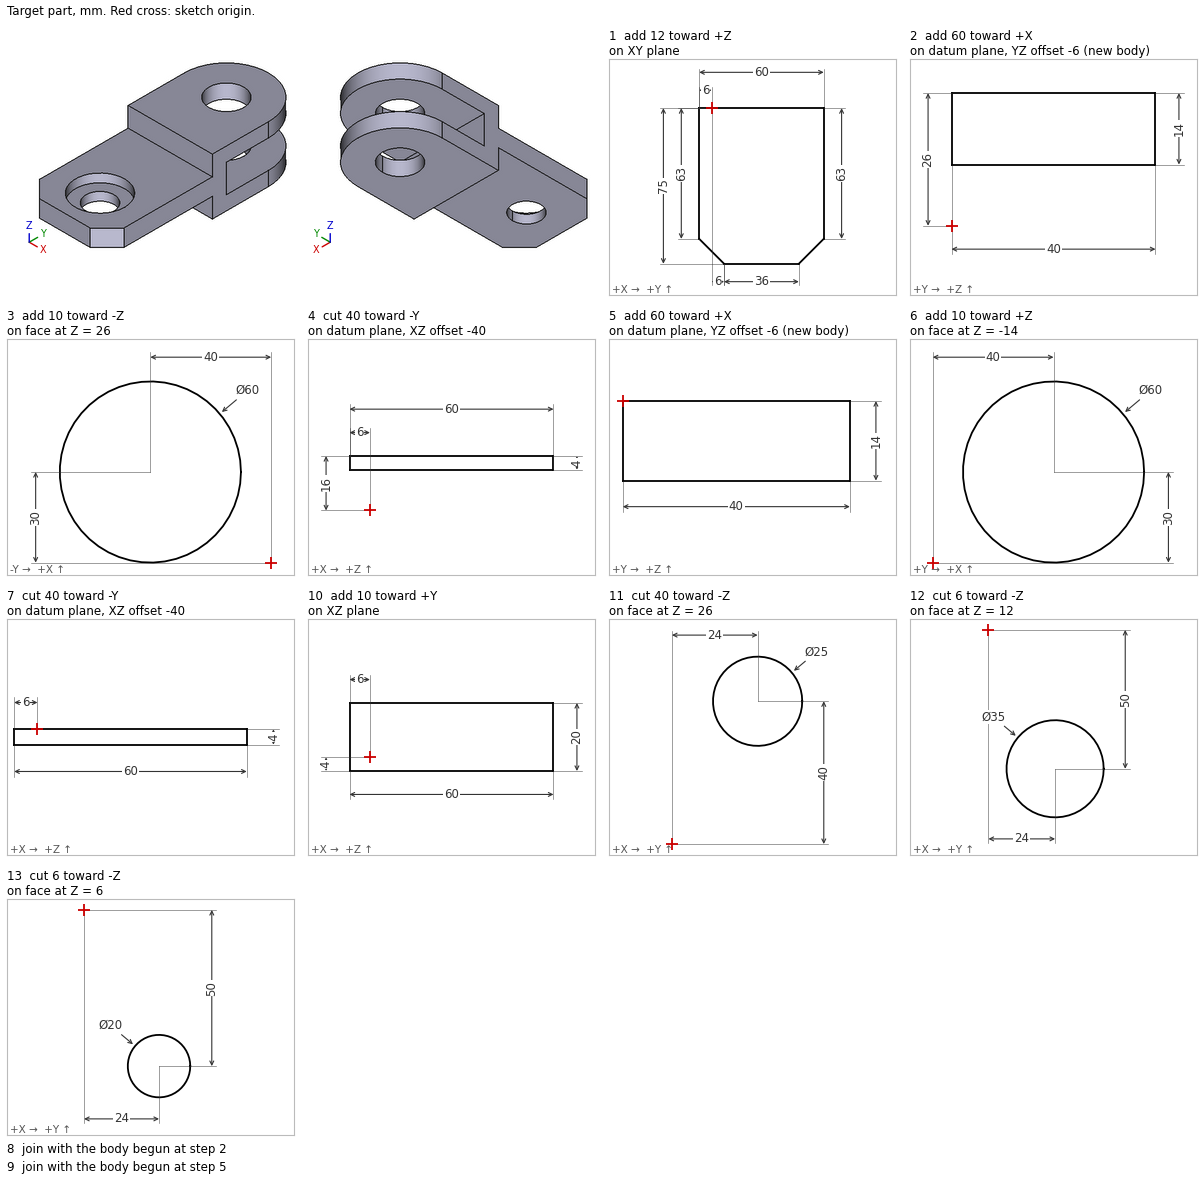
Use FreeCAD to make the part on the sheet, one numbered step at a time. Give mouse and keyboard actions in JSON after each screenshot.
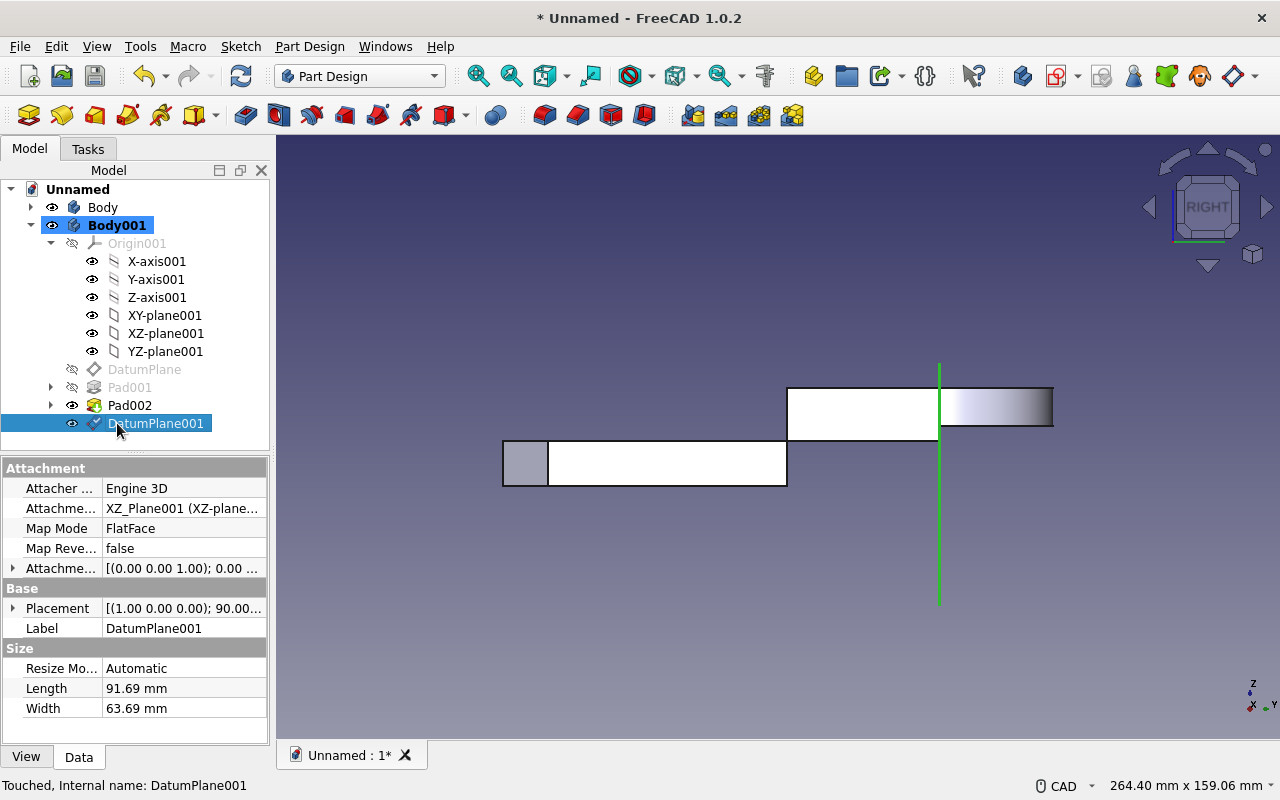
{"action": "left_click", "coordinate": [1056, 76]}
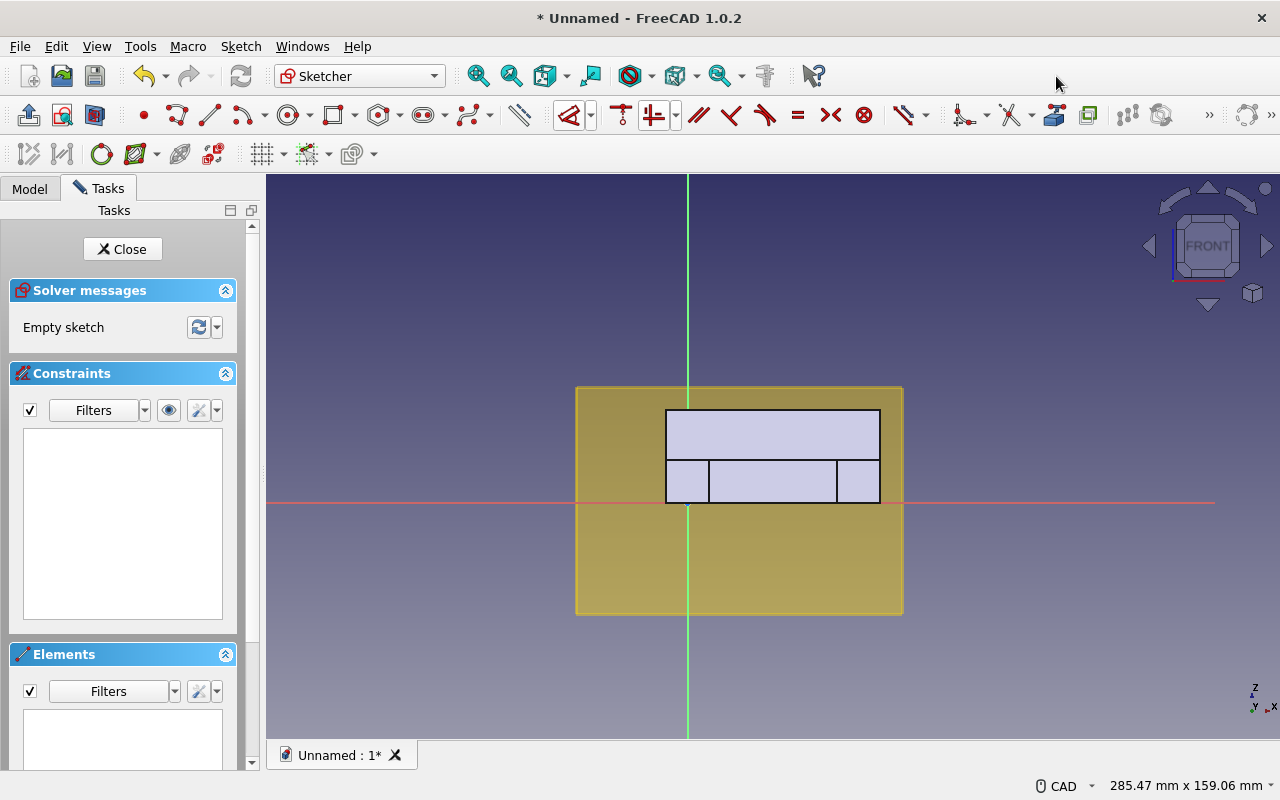
{"action": "left_click", "coordinate": [95, 116]}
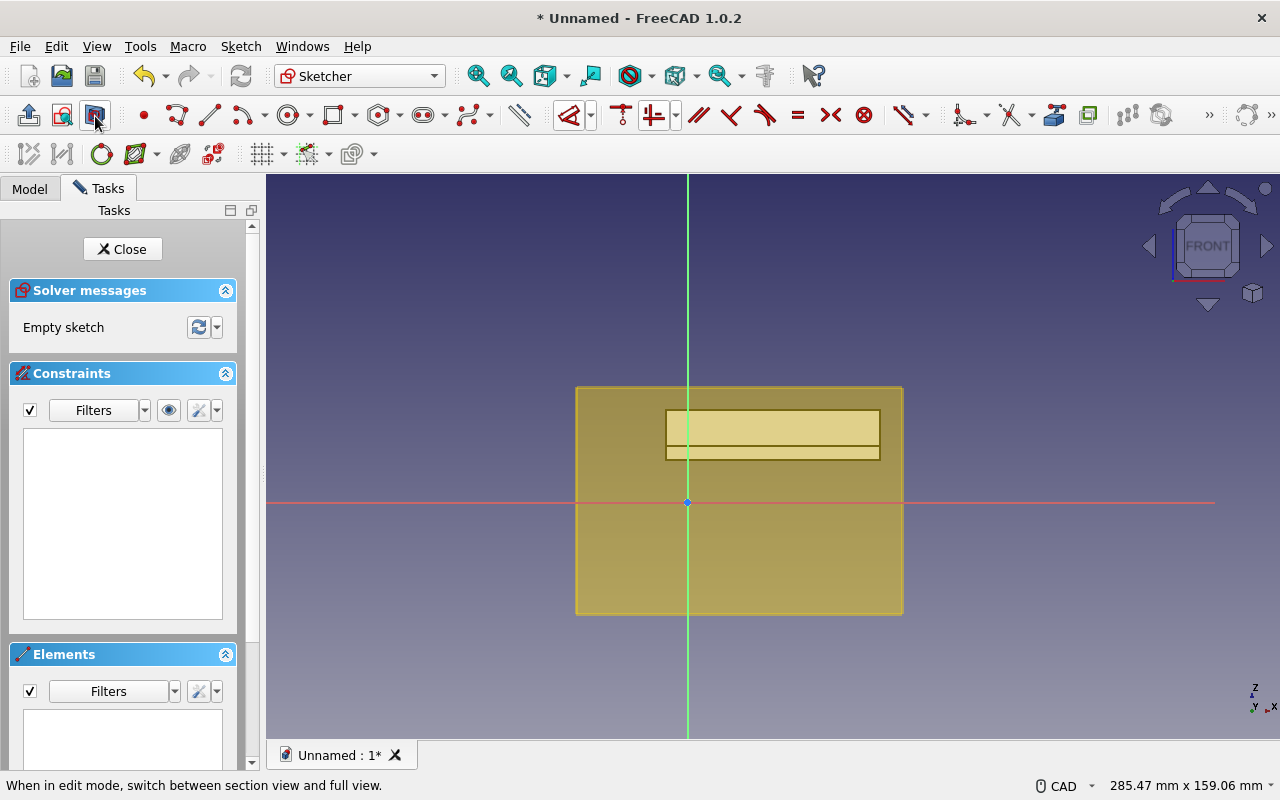
{"action": "scroll", "coordinate": [813, 485], "scroll_direction": "up", "scroll_amount": 5}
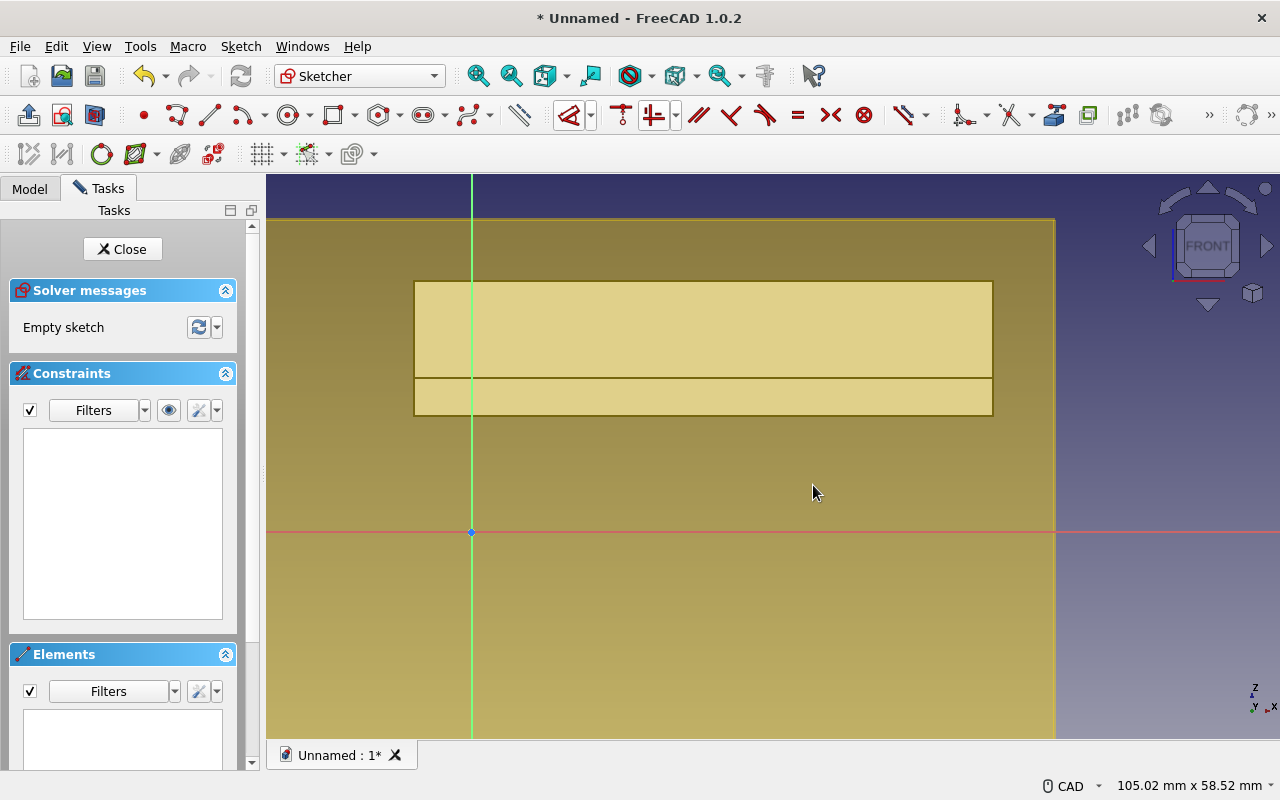
{"action": "left_click", "coordinate": [332, 116]}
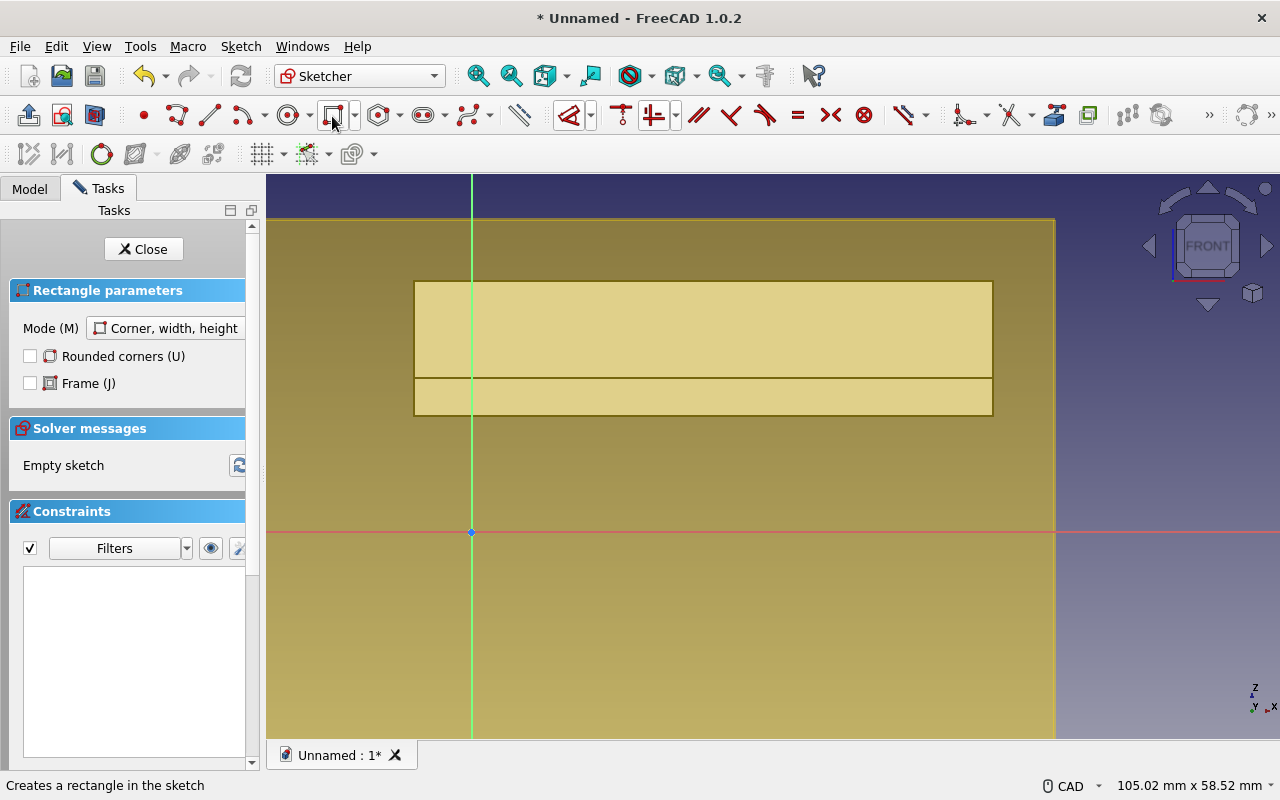
{"action": "left_click", "coordinate": [414, 378]}
{"action": "mouse_move", "coordinate": [993, 416]}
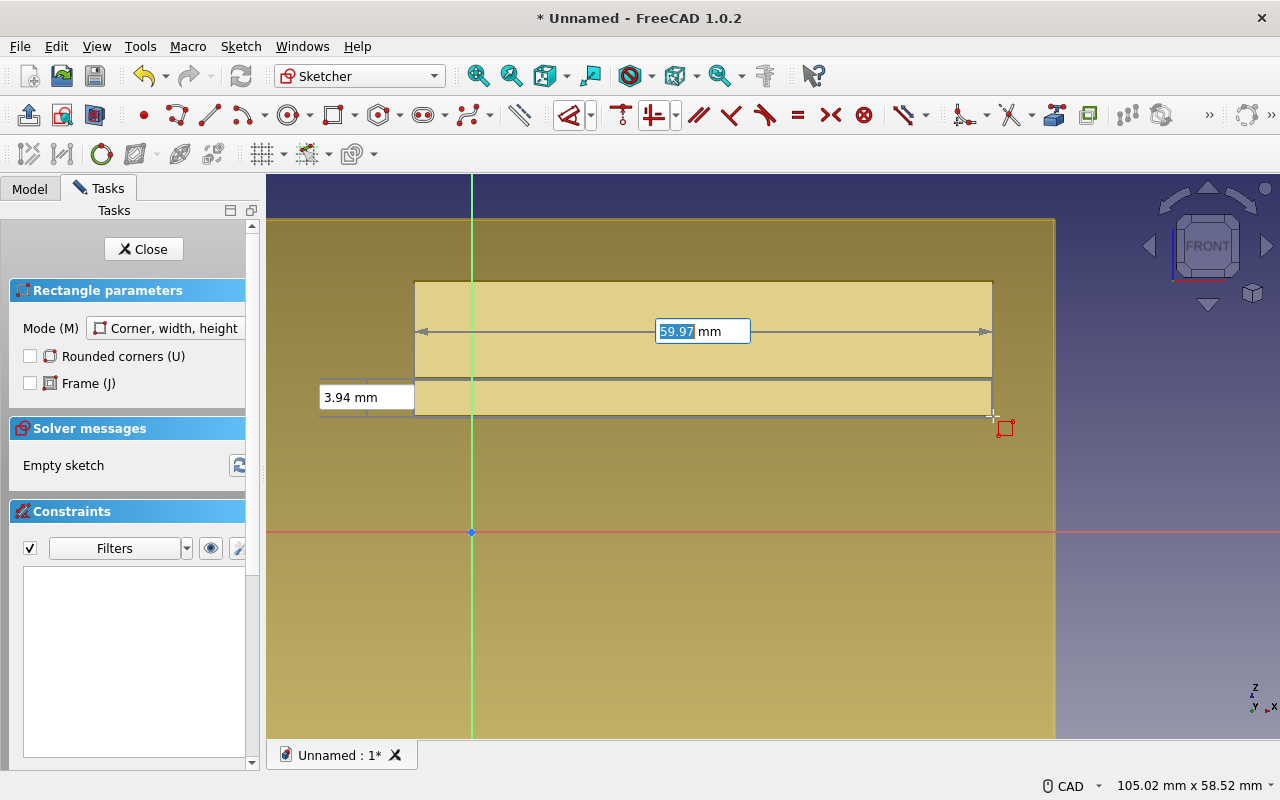
{"action": "type", "text": "60"}
{"action": "key", "text": "Tab"}
{"action": "type", "text": "4"}
{"action": "key", "text": "Return"}
{"action": "key", "text": "Escape"}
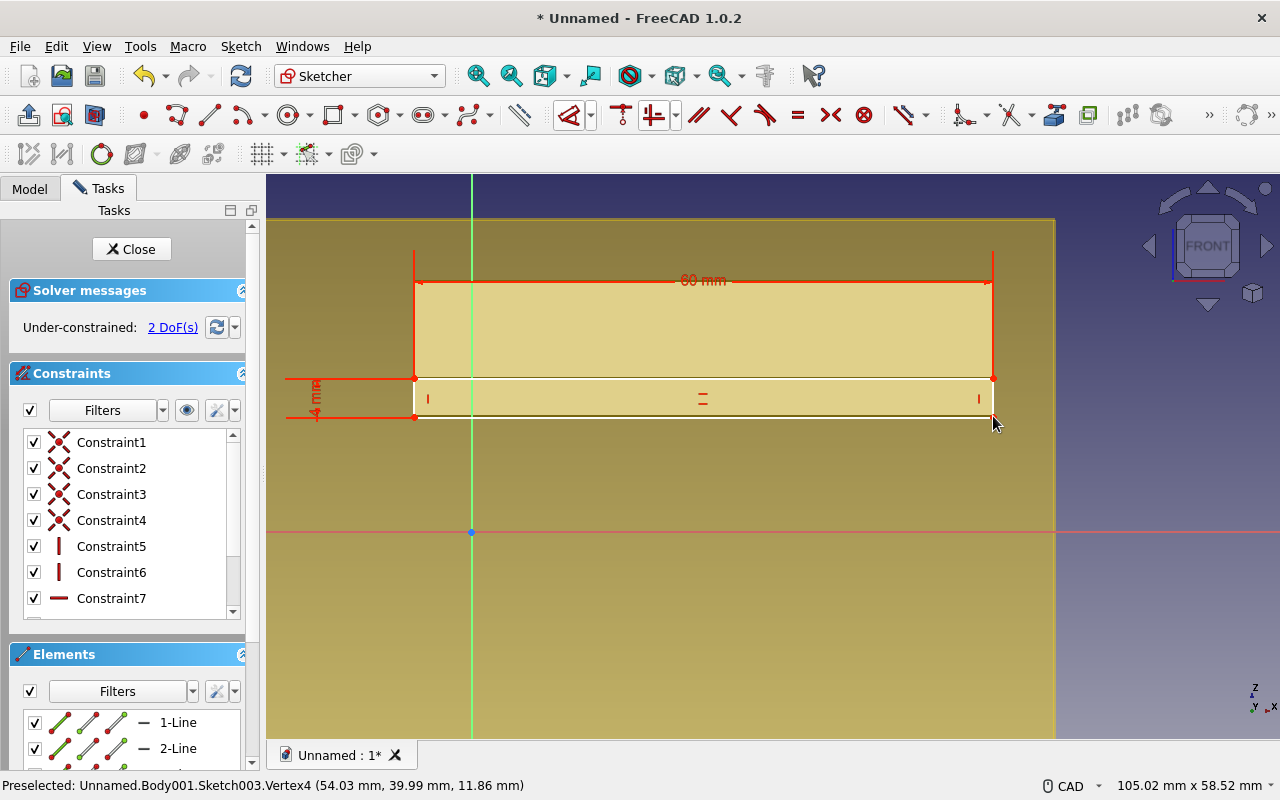
{"action": "left_click", "coordinate": [414, 379]}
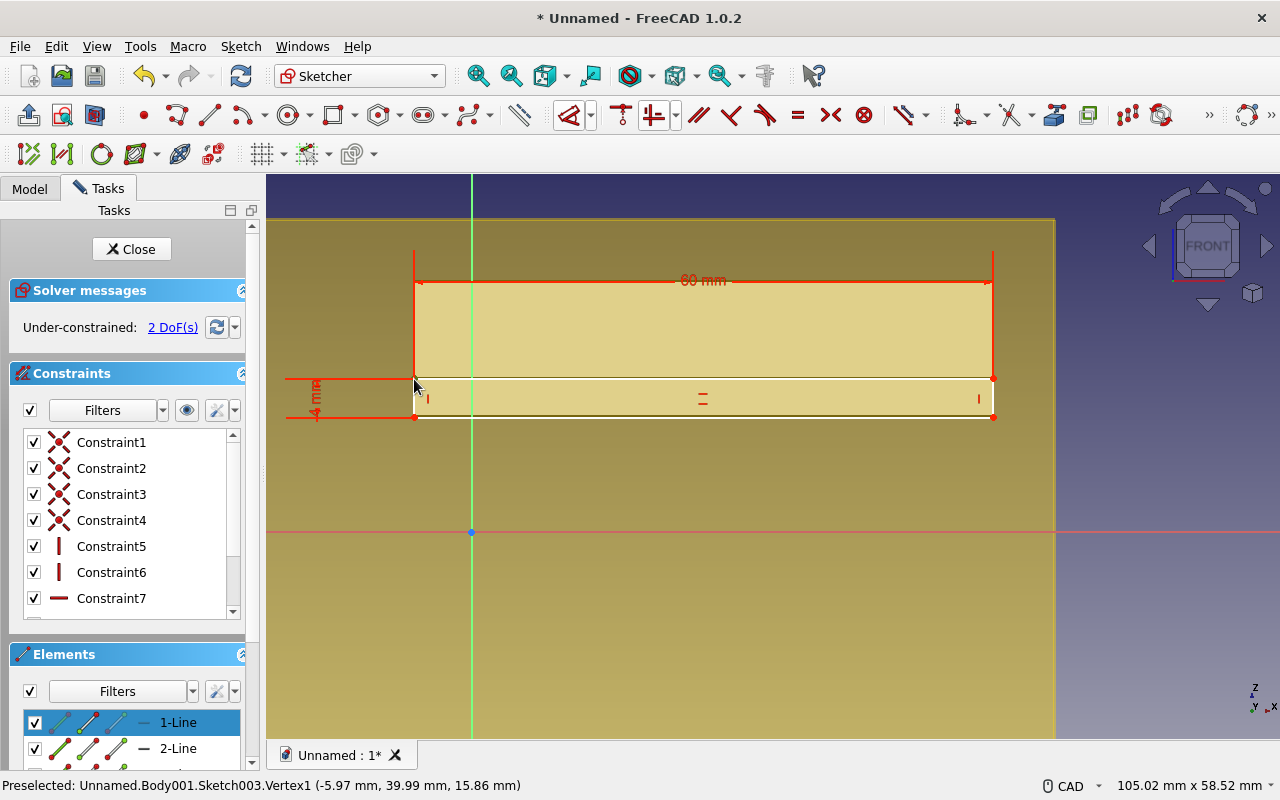
{"action": "key", "text": "l"}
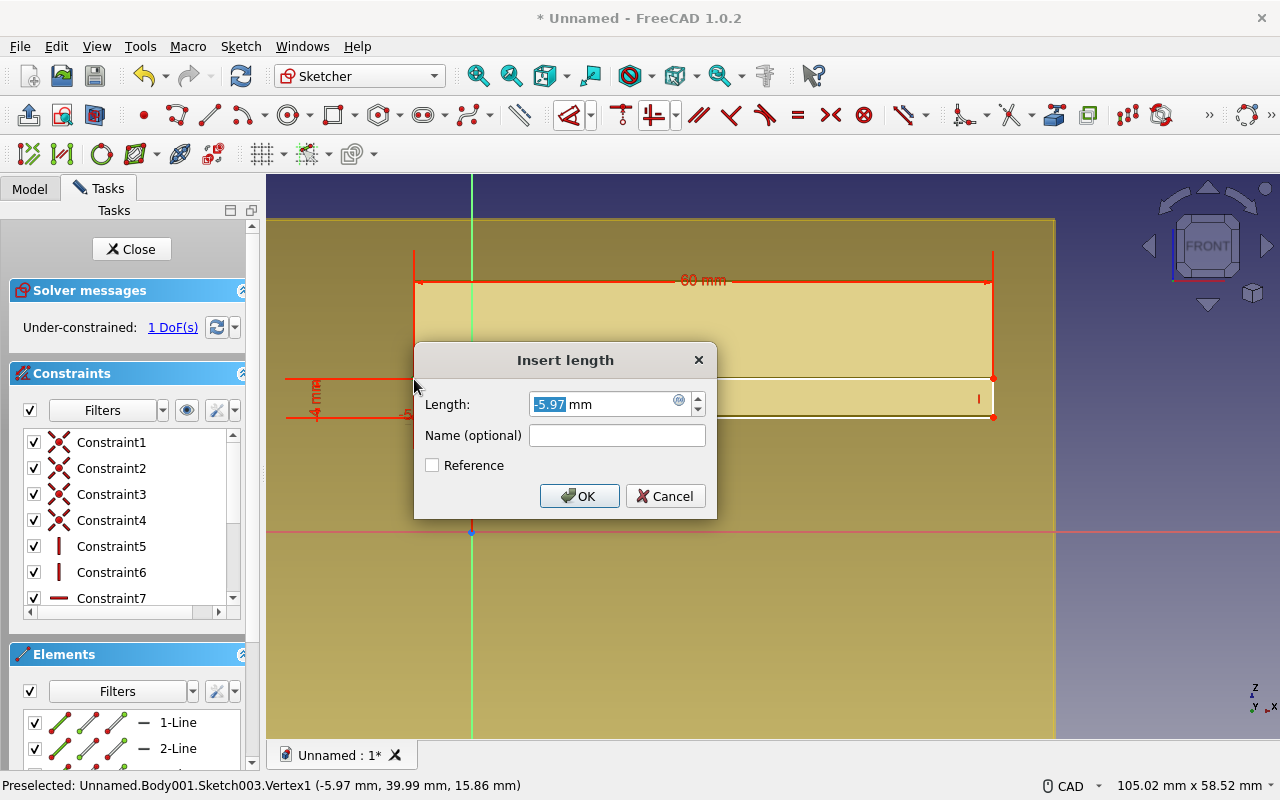
{"action": "type", "text": "-6"}
{"action": "key", "text": "Return"}